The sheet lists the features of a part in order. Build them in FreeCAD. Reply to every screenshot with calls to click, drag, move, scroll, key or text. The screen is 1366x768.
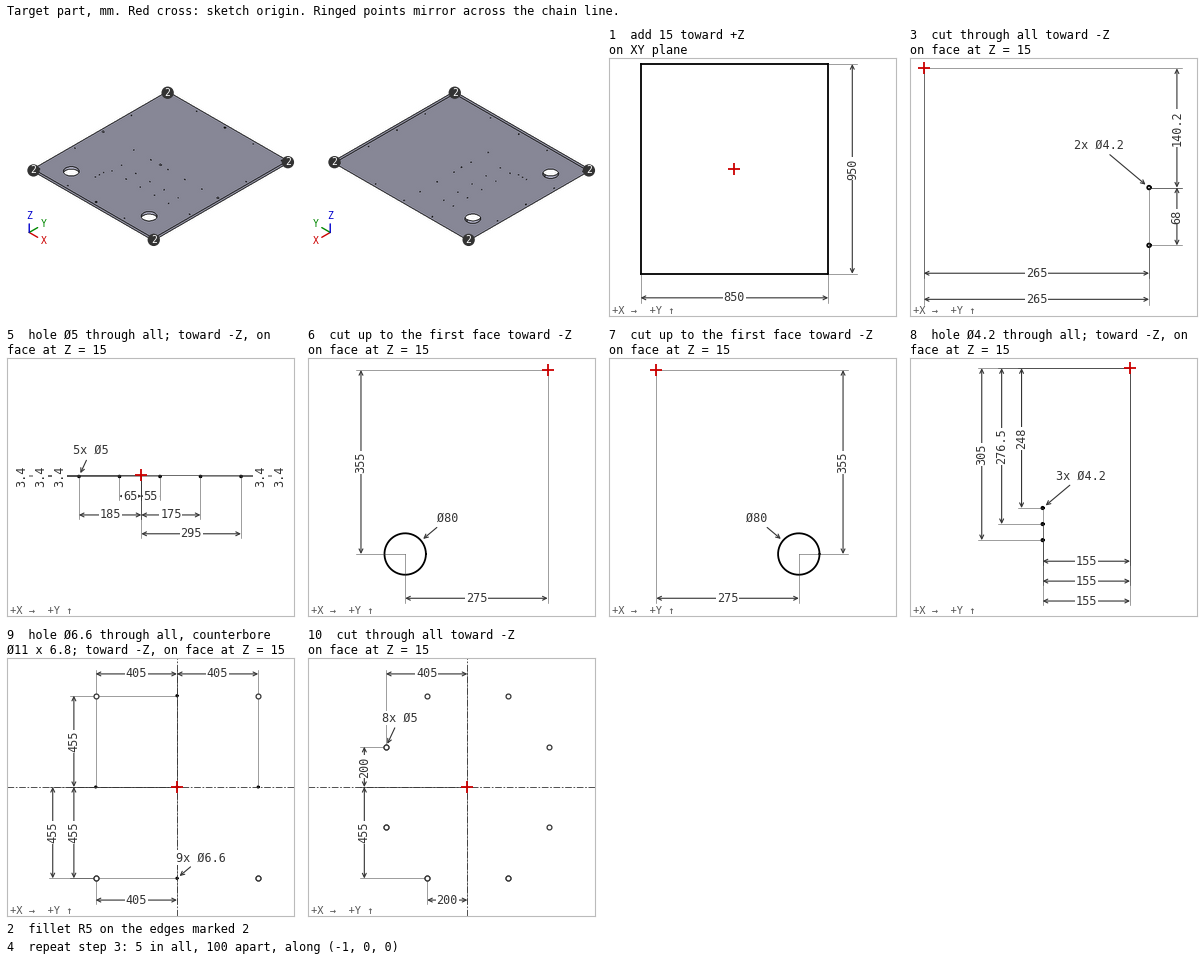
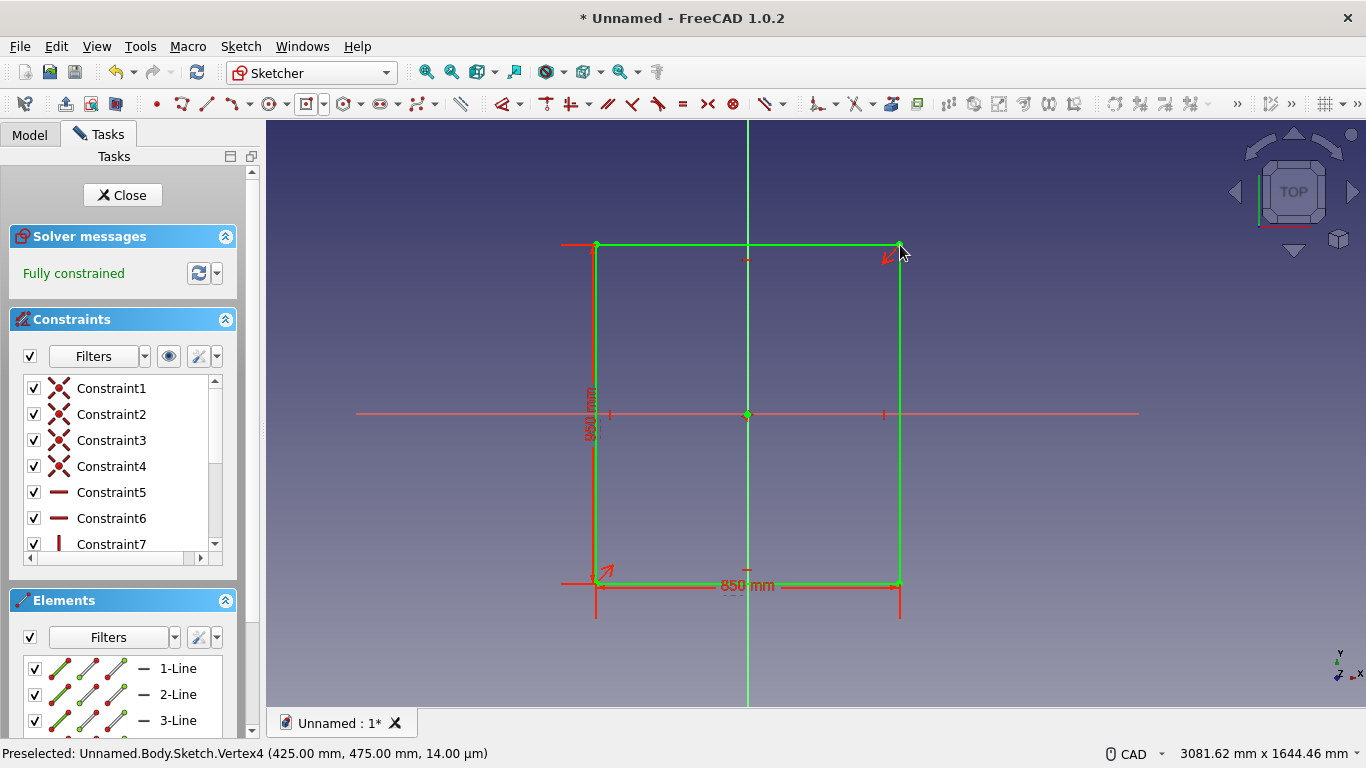
click(123, 195)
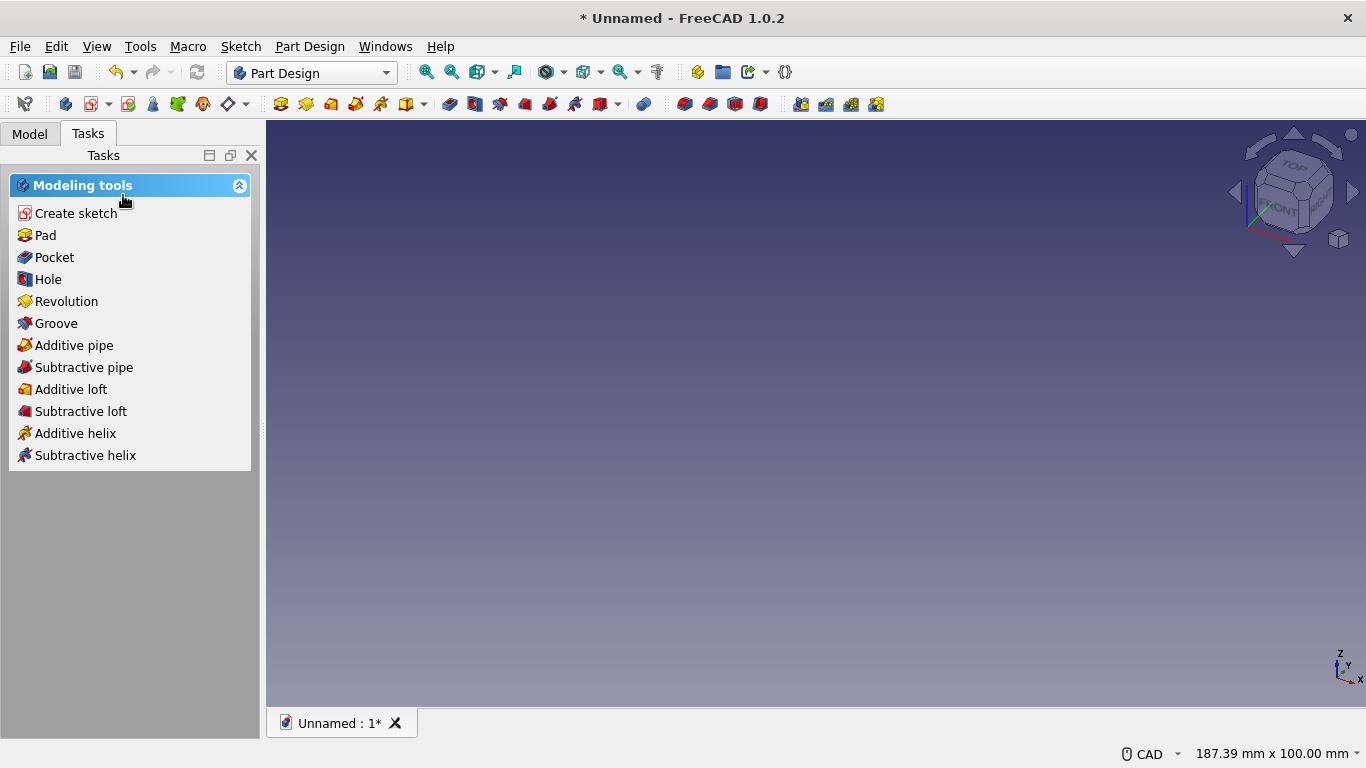
click(281, 104)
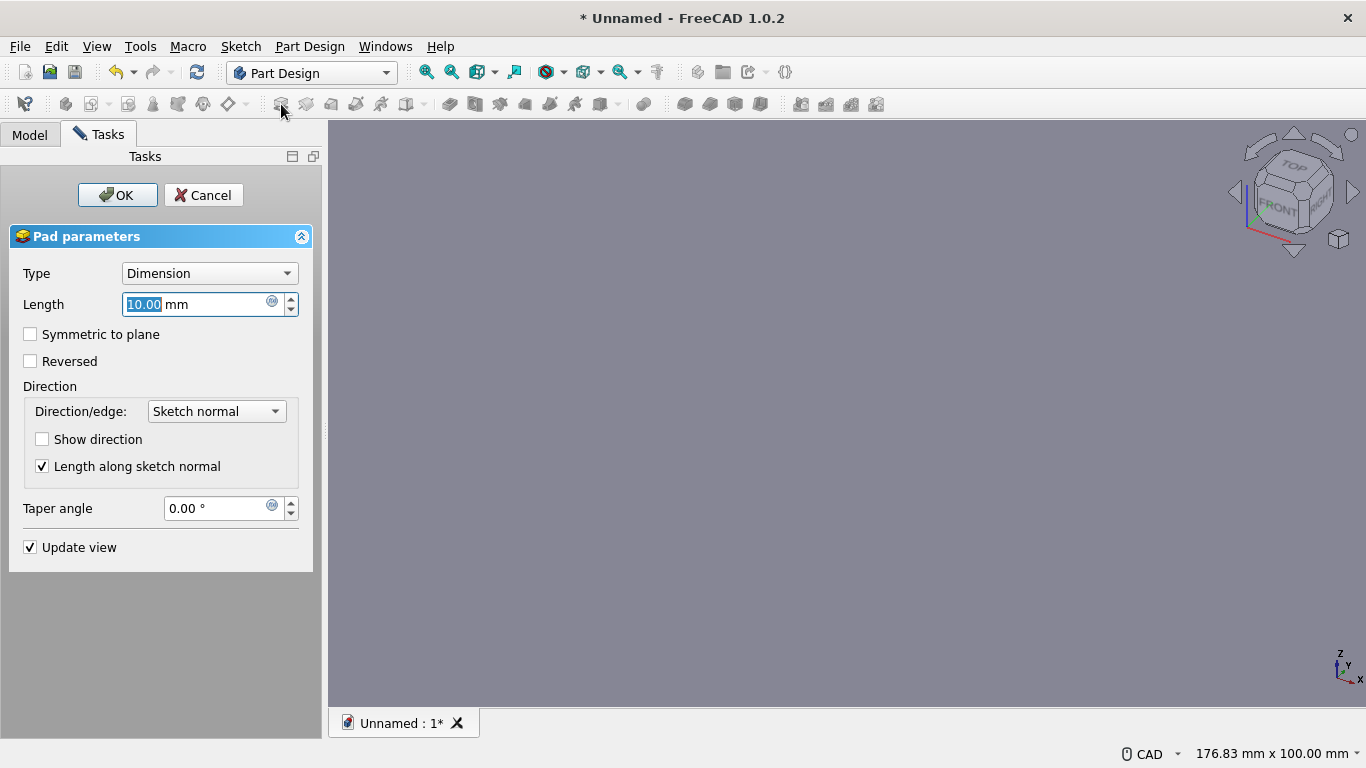
text(15)
key(Tab)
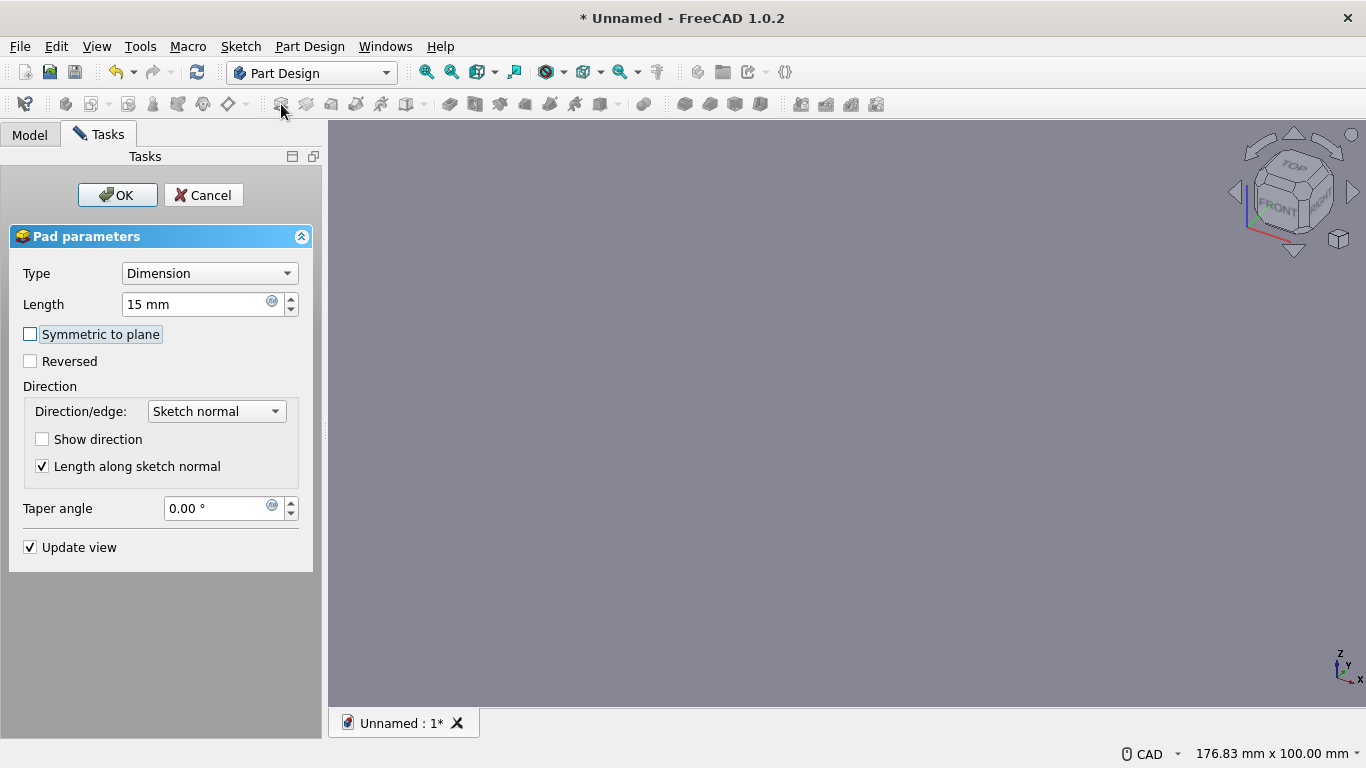
click(118, 195)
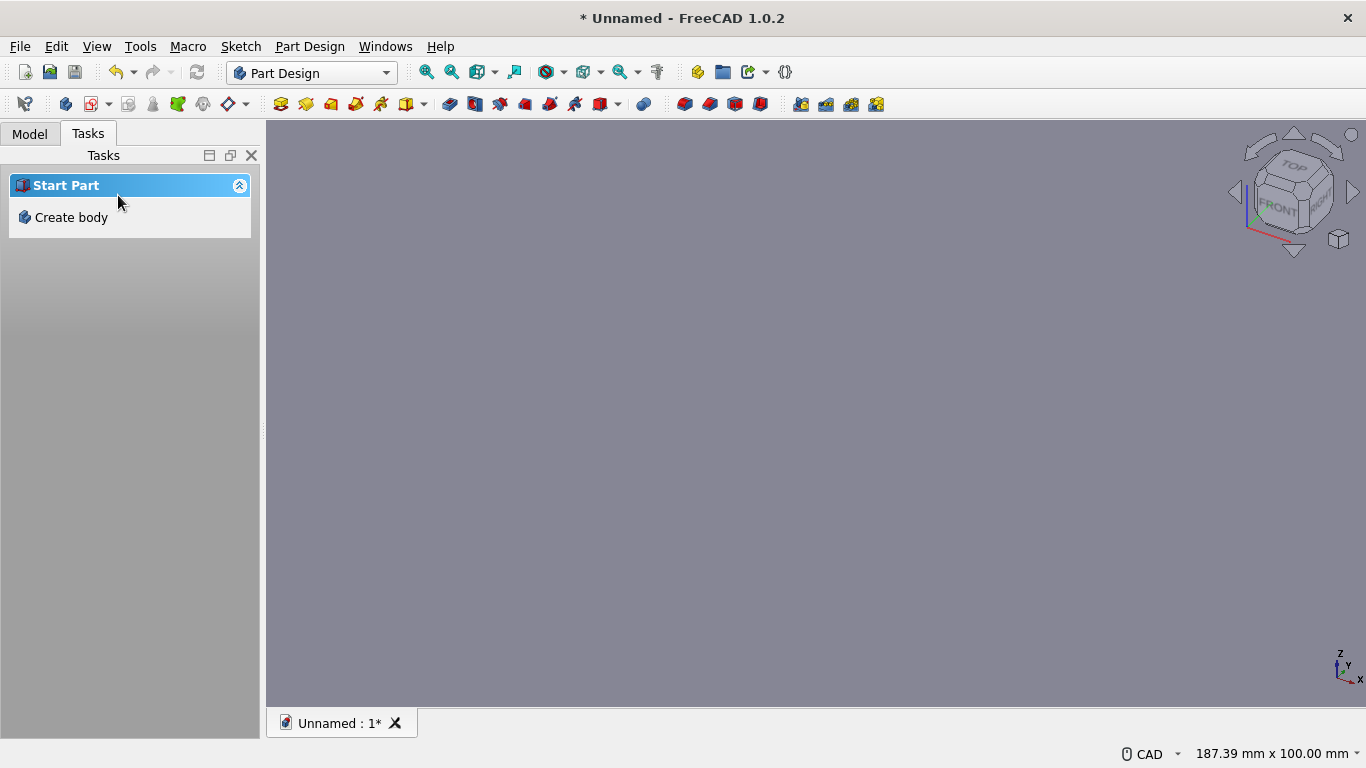
click(427, 72)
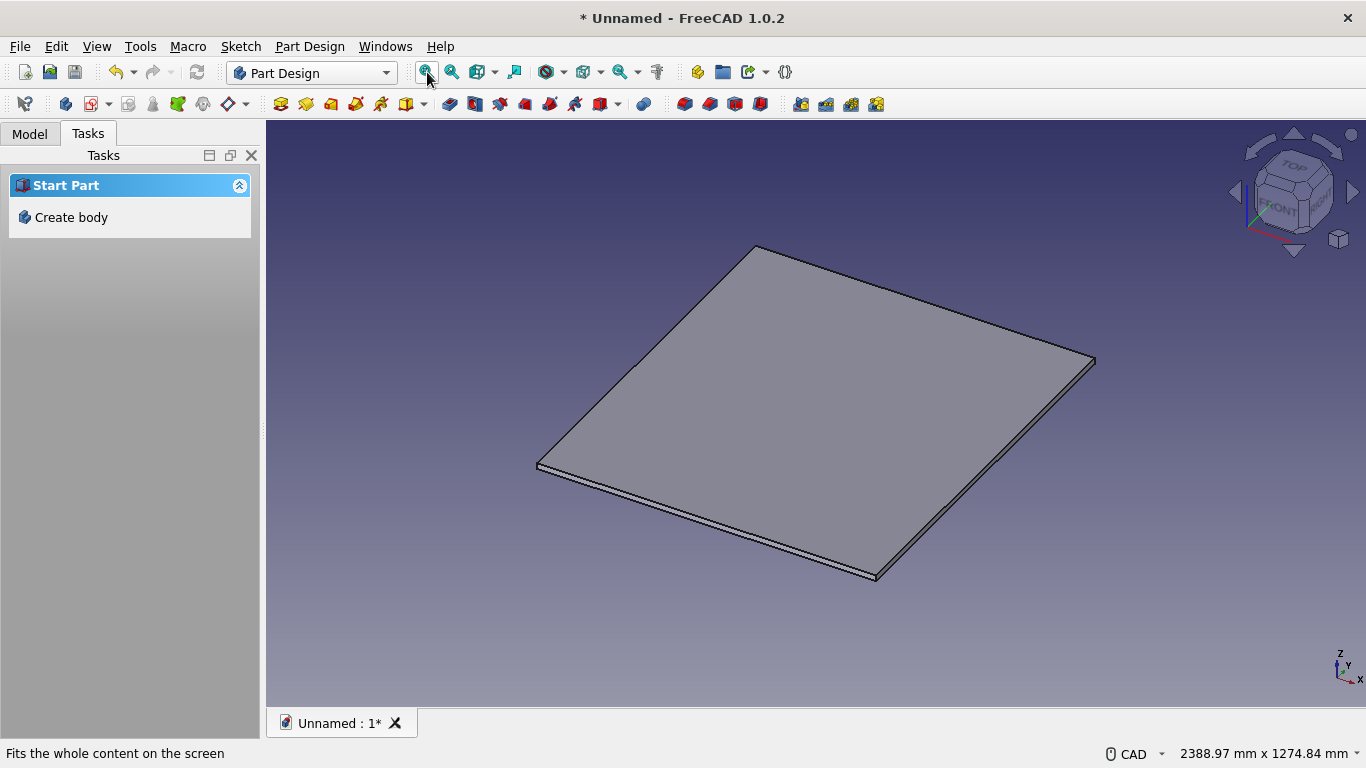
scroll(756, 248, up, 9)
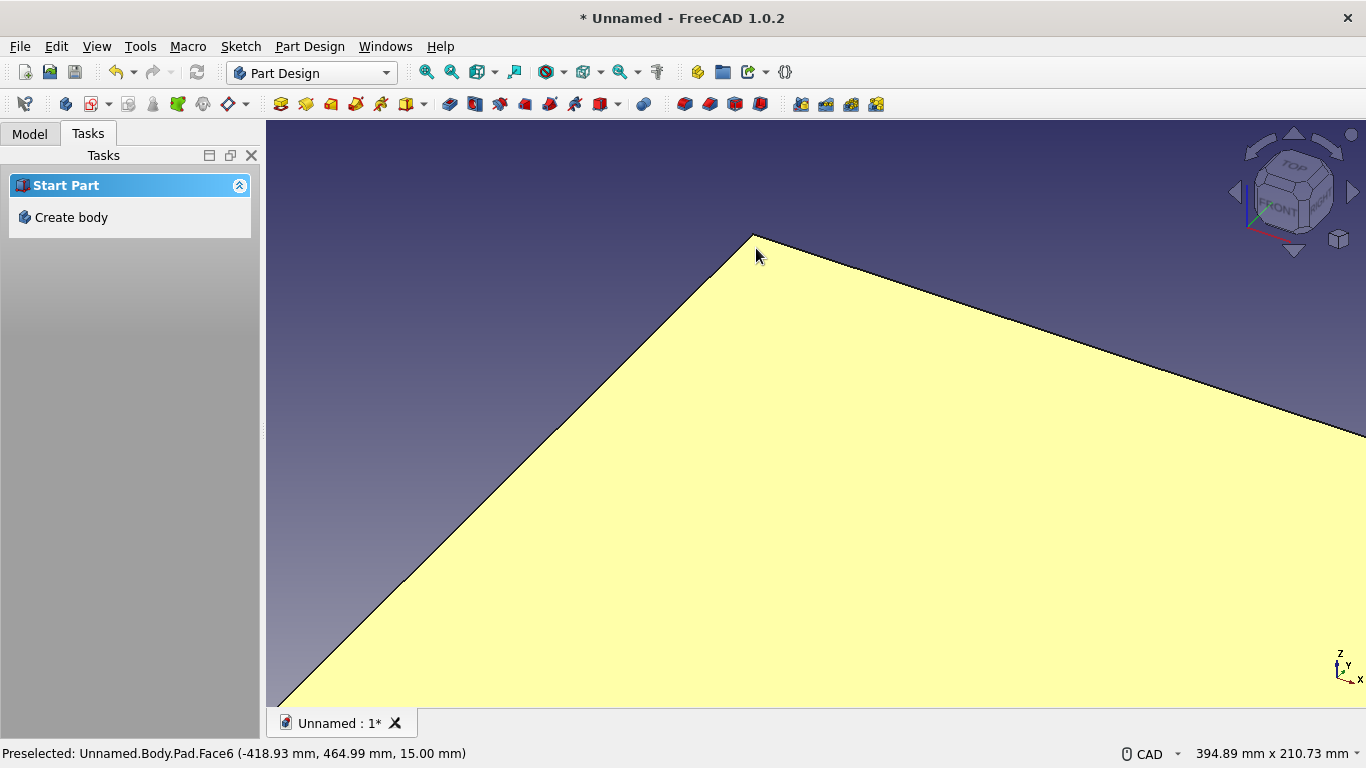
click(427, 72)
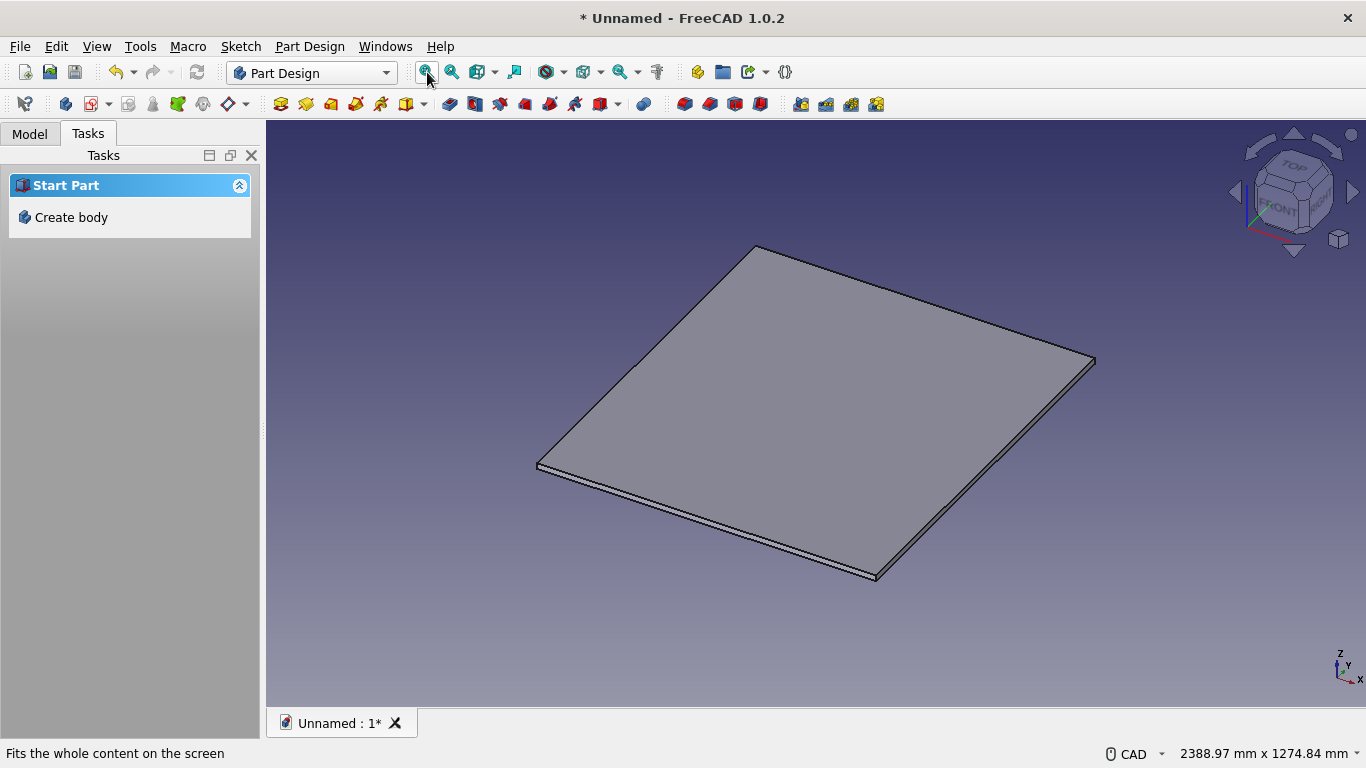
key(0)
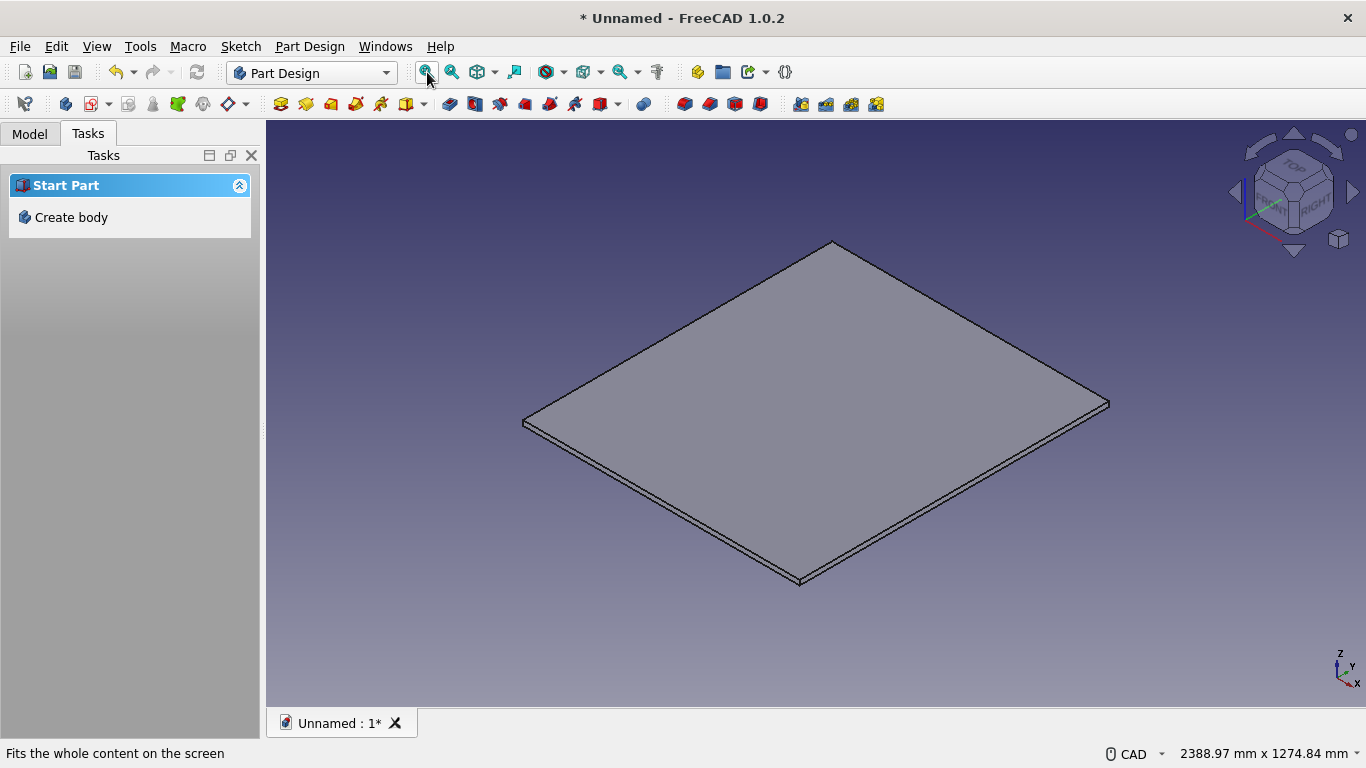
scroll(832, 243, up, 9)